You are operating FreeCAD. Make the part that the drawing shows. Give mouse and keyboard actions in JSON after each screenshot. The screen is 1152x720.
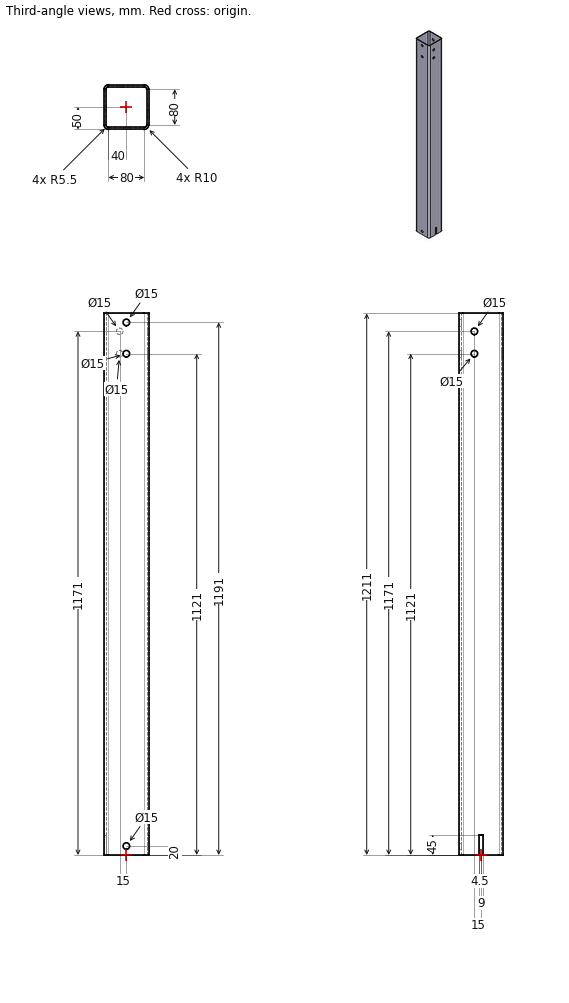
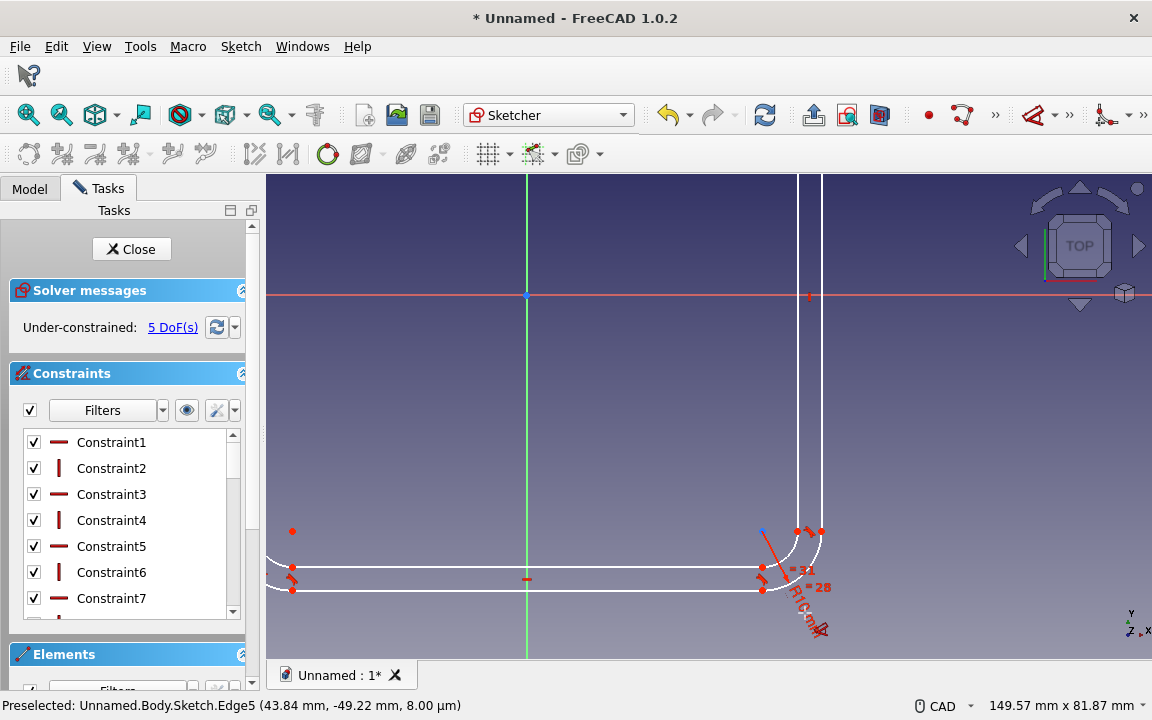
{"action": "scroll", "coordinate": [779, 564], "scroll_direction": "down", "scroll_amount": 3}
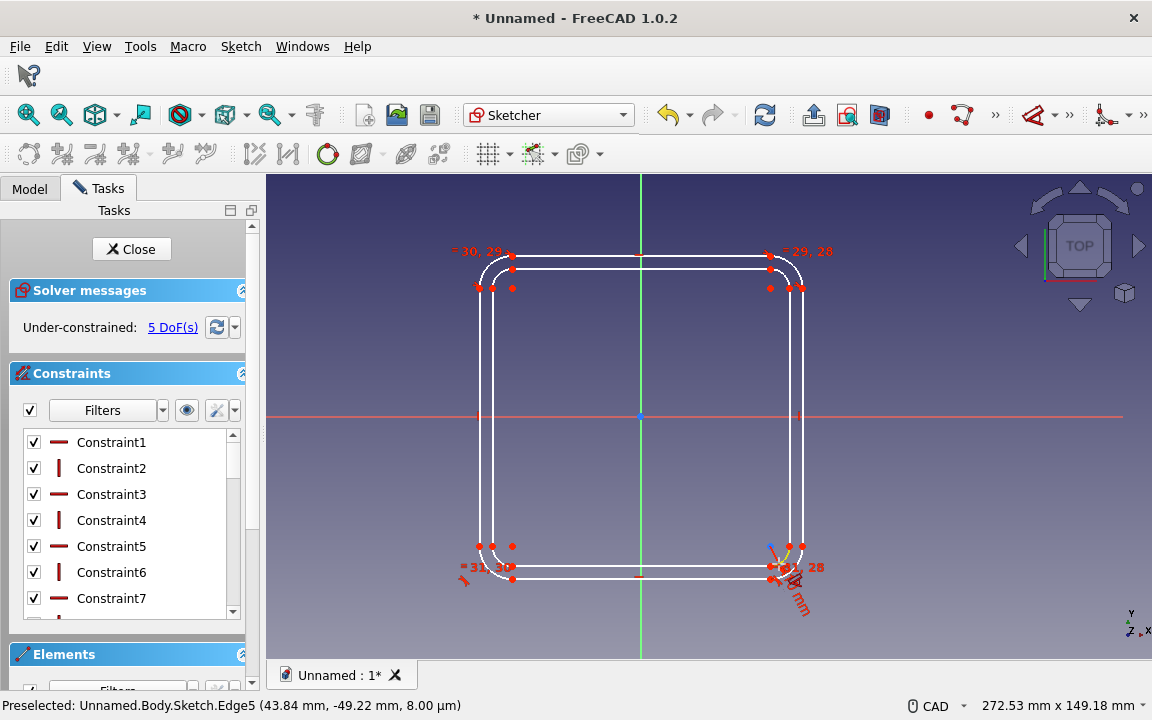
{"action": "scroll", "coordinate": [495, 555], "scroll_direction": "up", "scroll_amount": 4}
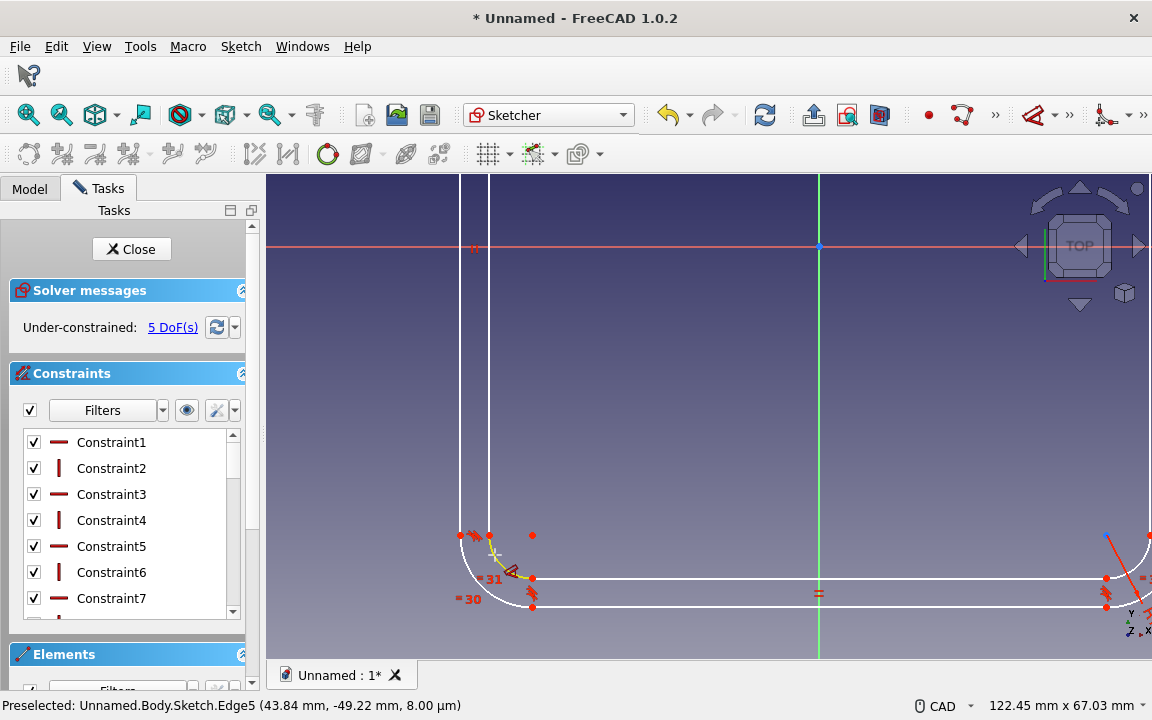
{"action": "left_click", "coordinate": [494, 555]}
{"action": "left_click", "coordinate": [600, 501]}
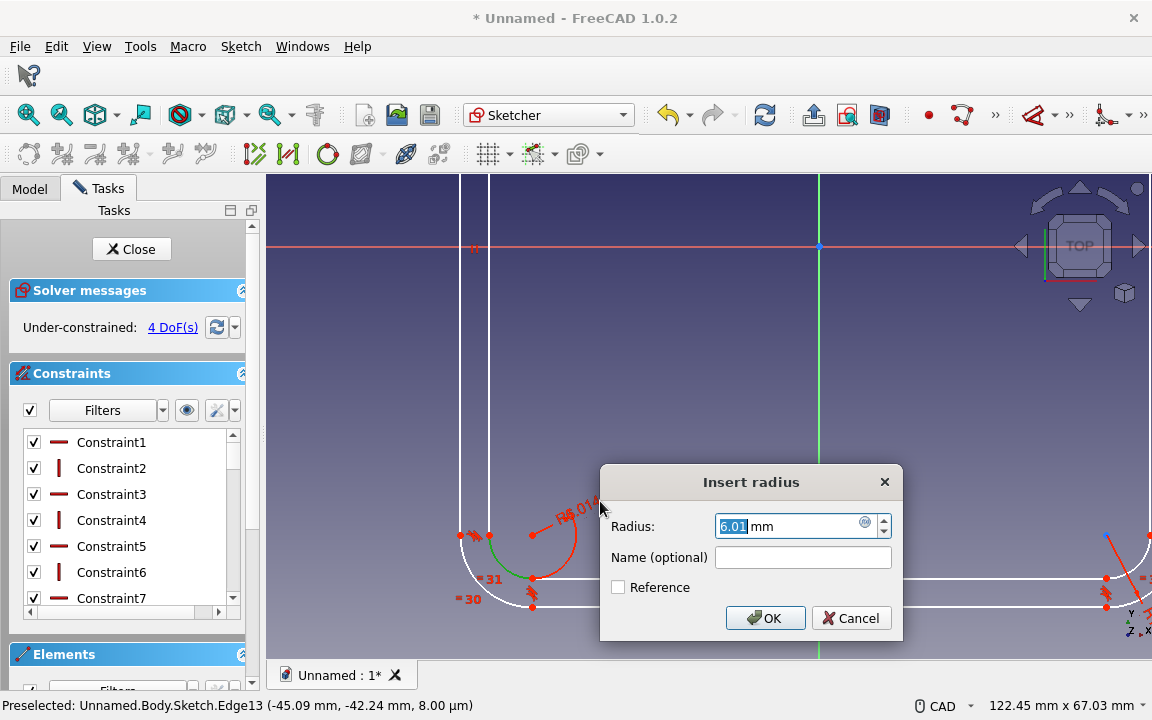
{"action": "type", "text": "5.5"}
{"action": "key", "text": "Return"}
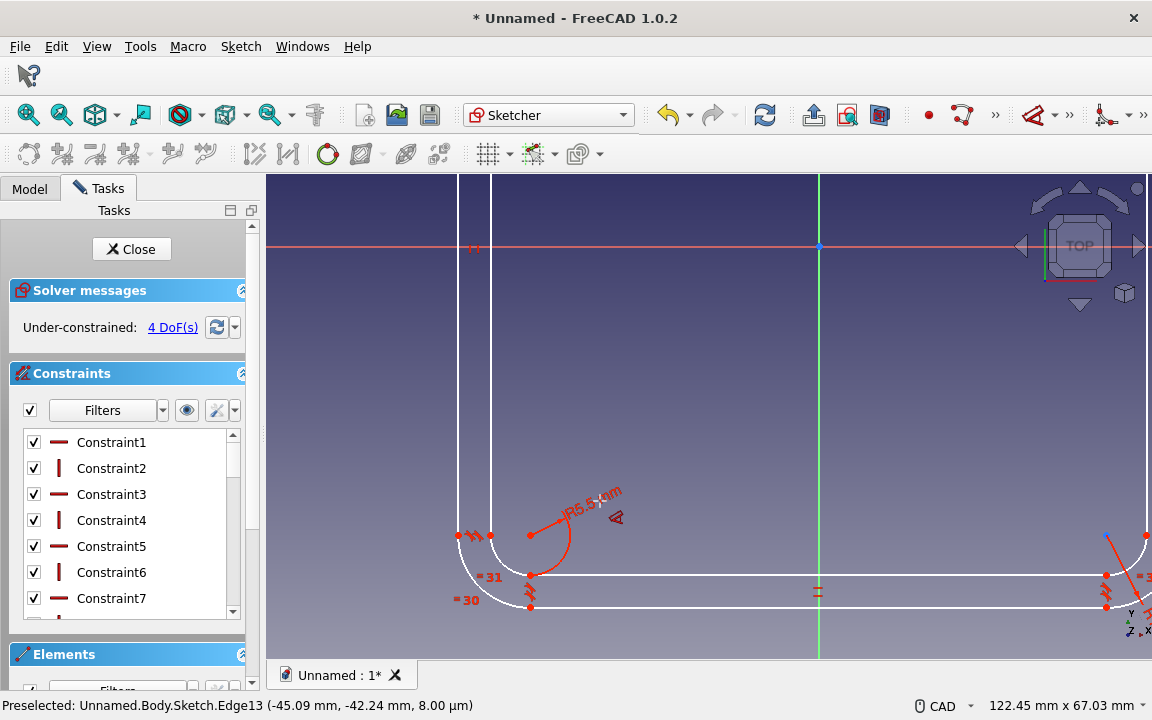
{"action": "left_click", "coordinate": [703, 608]}
{"action": "left_click", "coordinate": [759, 550]}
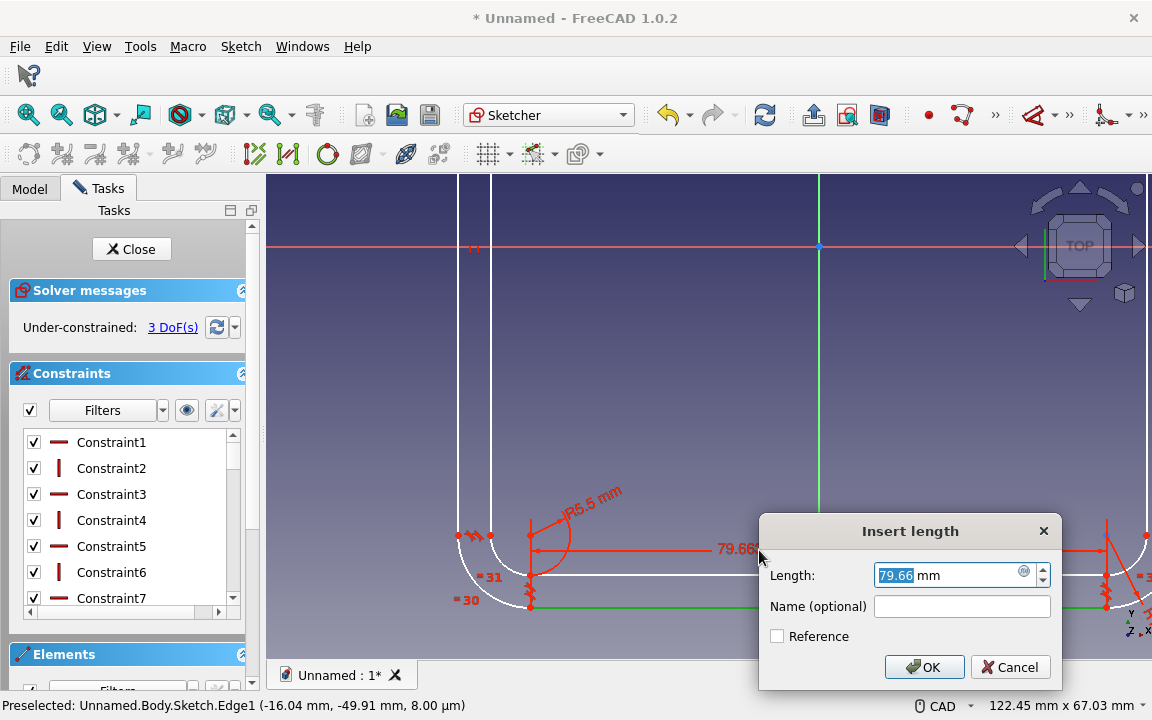
{"action": "type", "text": "80"}
{"action": "key", "text": "Return"}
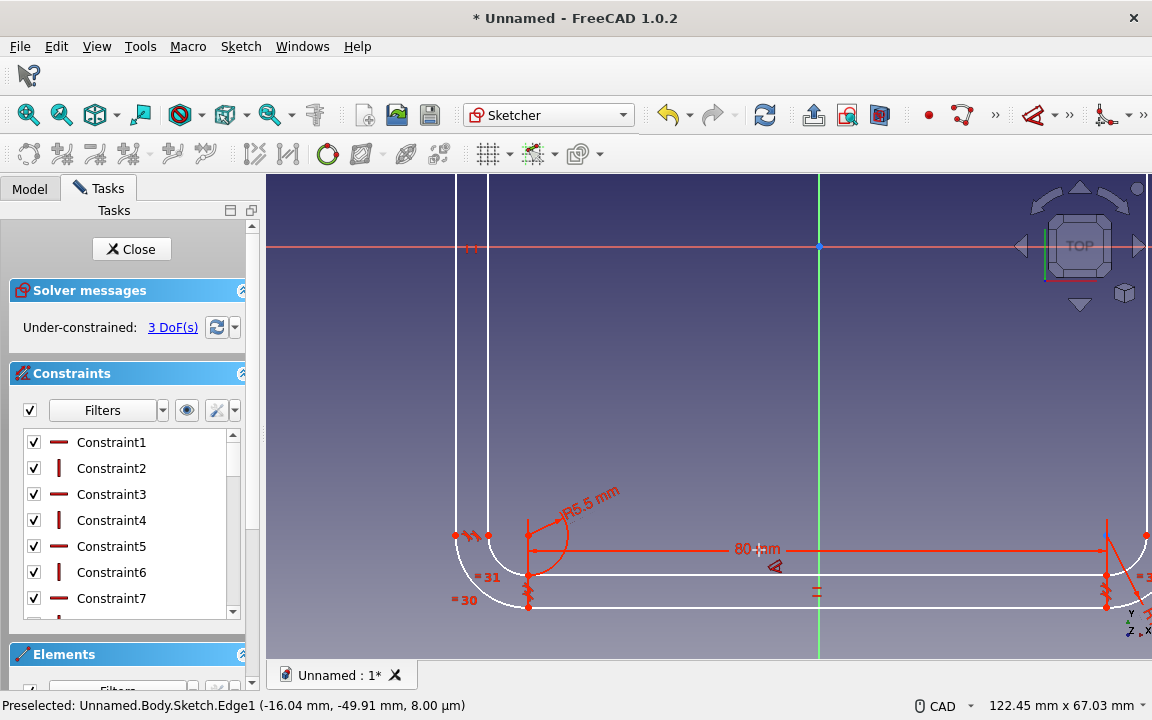
{"action": "scroll", "coordinate": [495, 555], "scroll_direction": "down", "scroll_amount": 4}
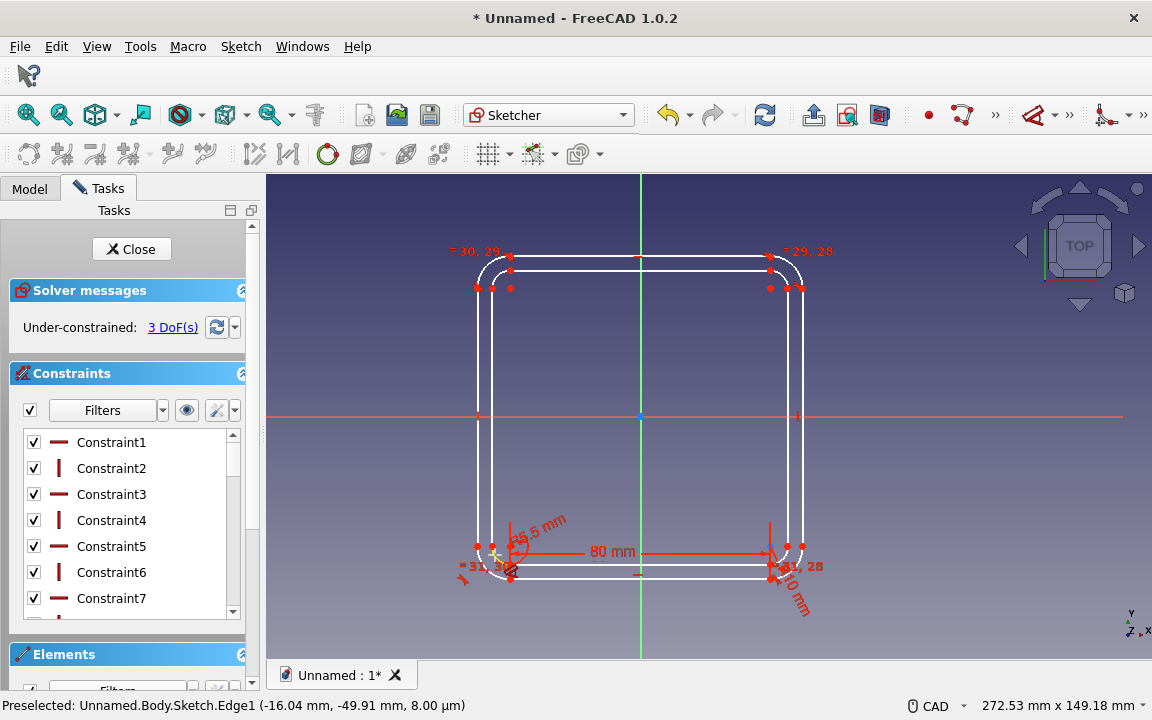
{"action": "left_click", "coordinate": [803, 469]}
{"action": "left_click", "coordinate": [837, 358]}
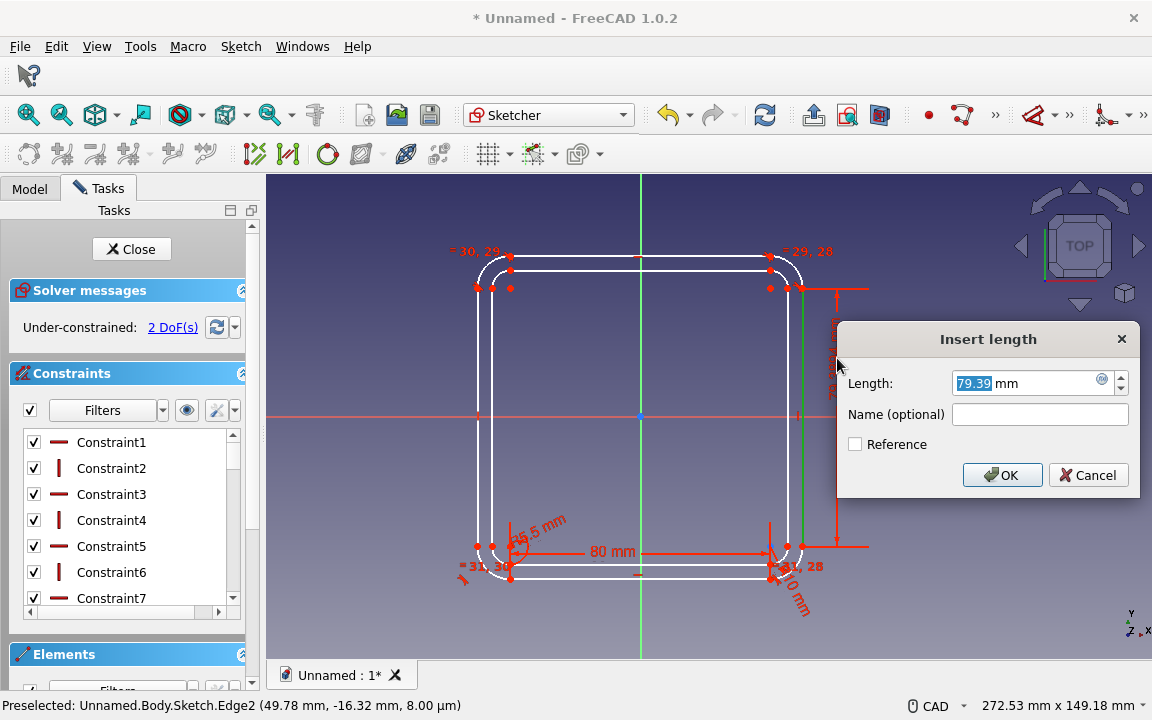
{"action": "type", "text": "80"}
{"action": "key", "text": "Return"}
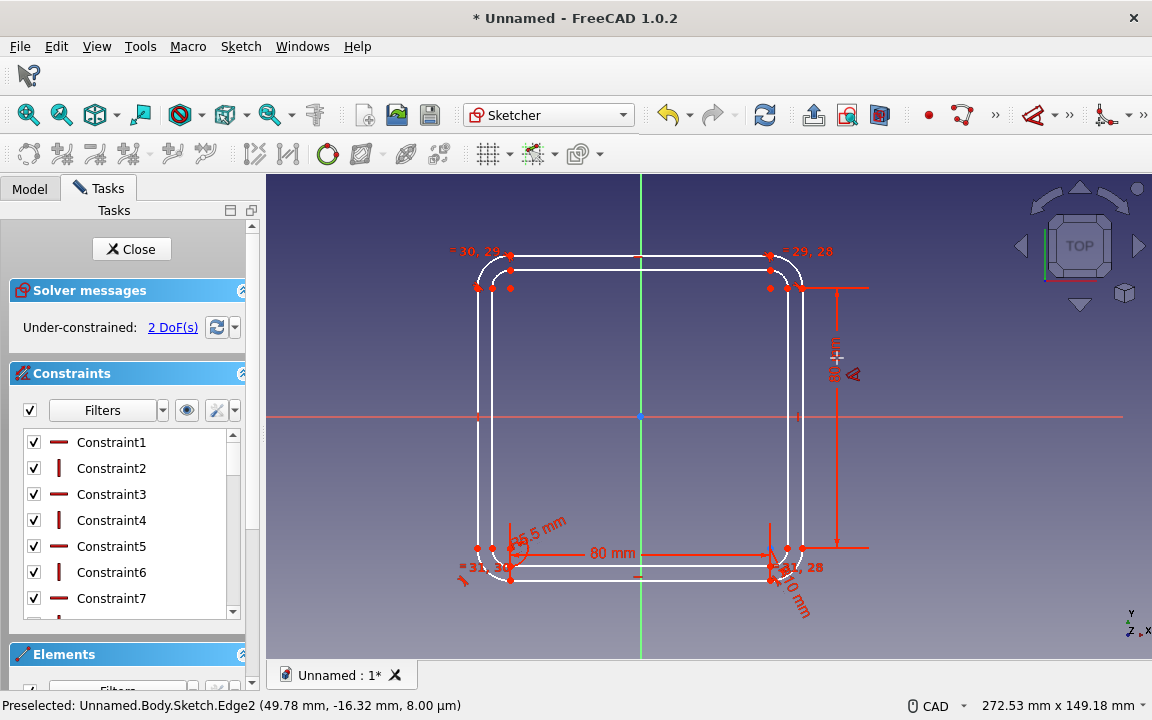
{"action": "left_click", "coordinate": [510, 581]}
{"action": "left_click", "coordinate": [575, 615]}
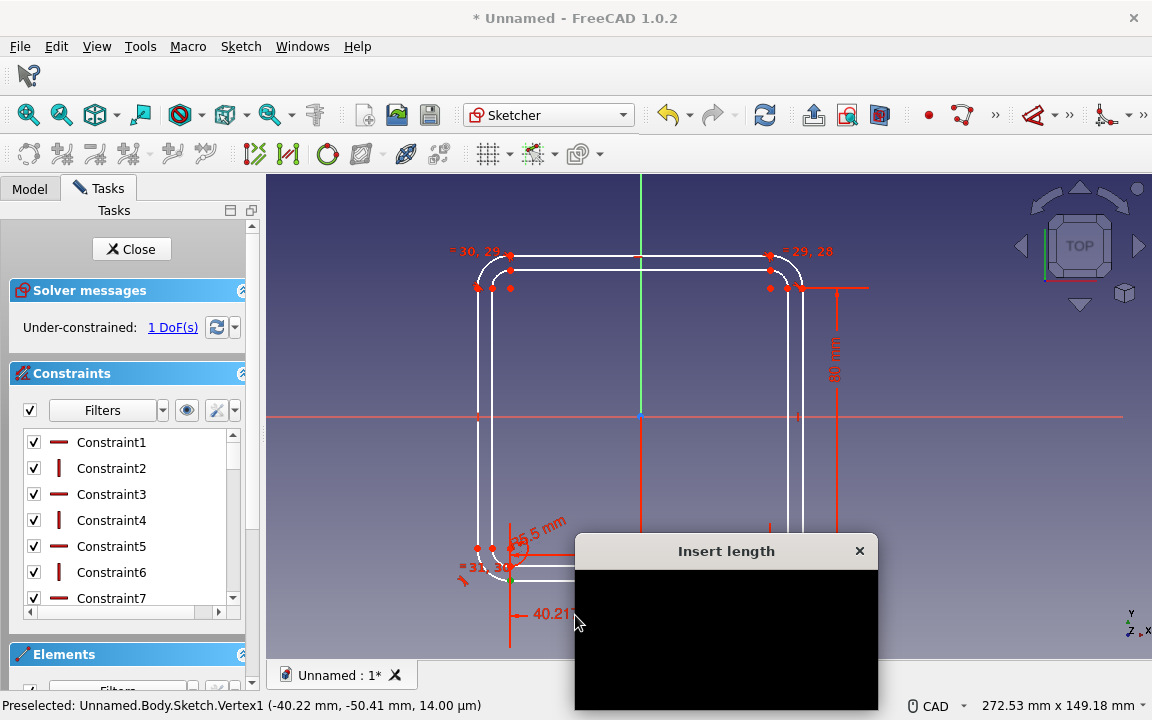
{"action": "type", "text": "40"}
{"action": "key", "text": "Return"}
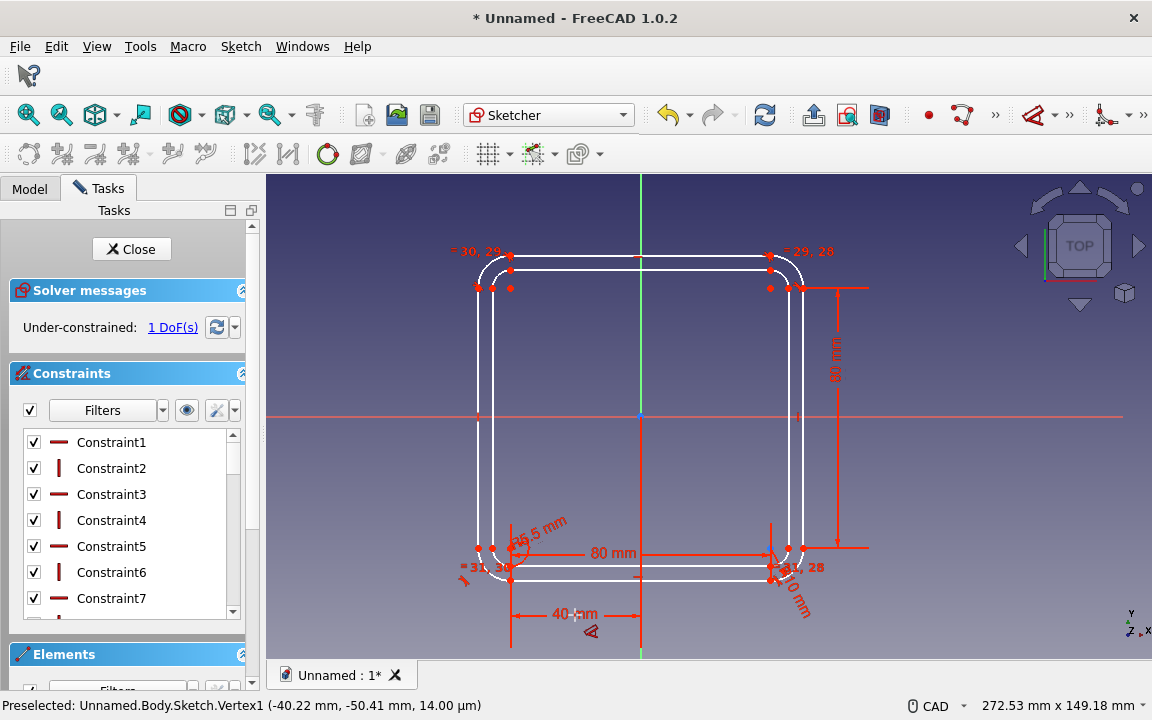
{"action": "left_click", "coordinate": [511, 581]}
{"action": "left_click", "coordinate": [675, 499]}